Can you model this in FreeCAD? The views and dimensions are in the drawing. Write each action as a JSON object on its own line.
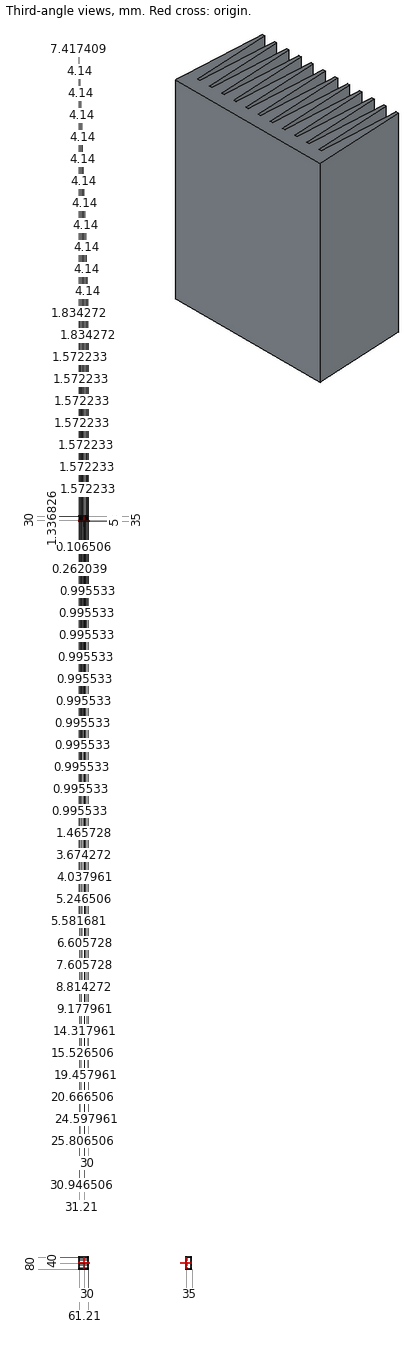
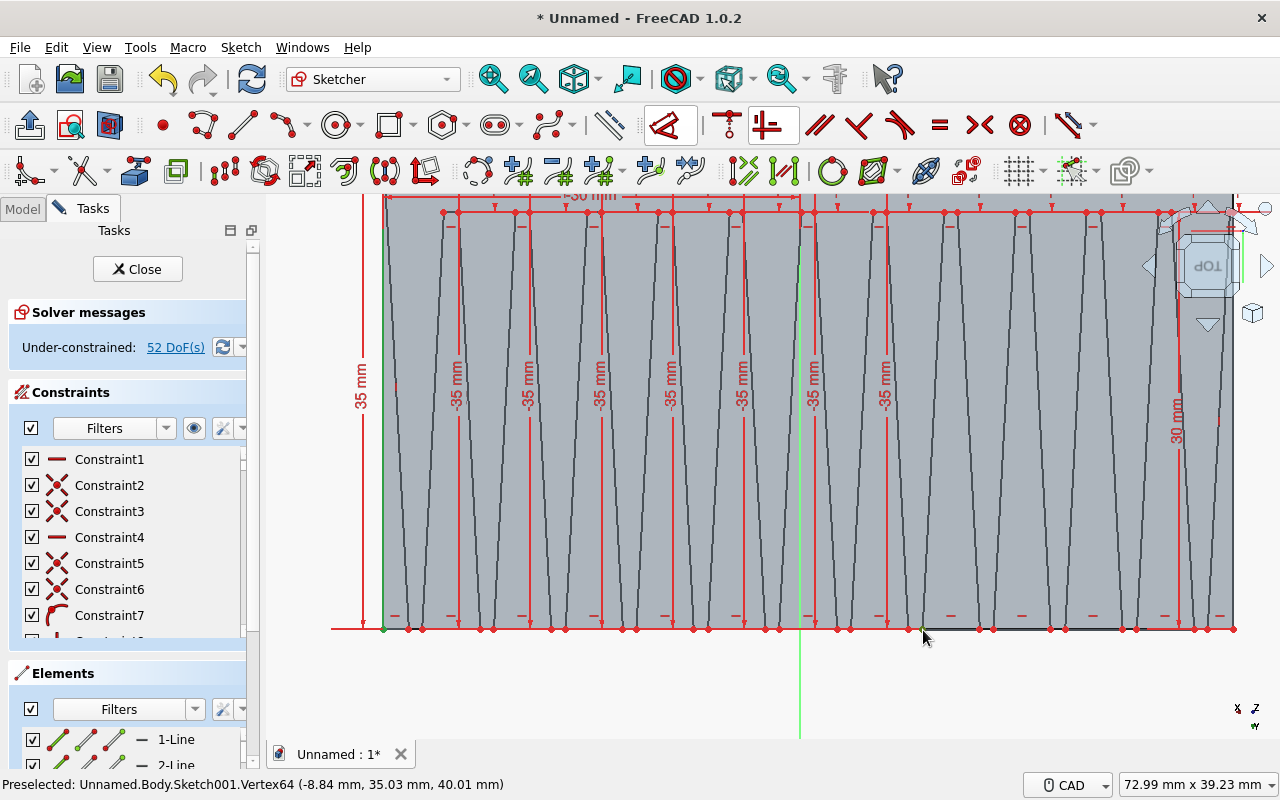
{"action": "left_click", "coordinate": [692, 126]}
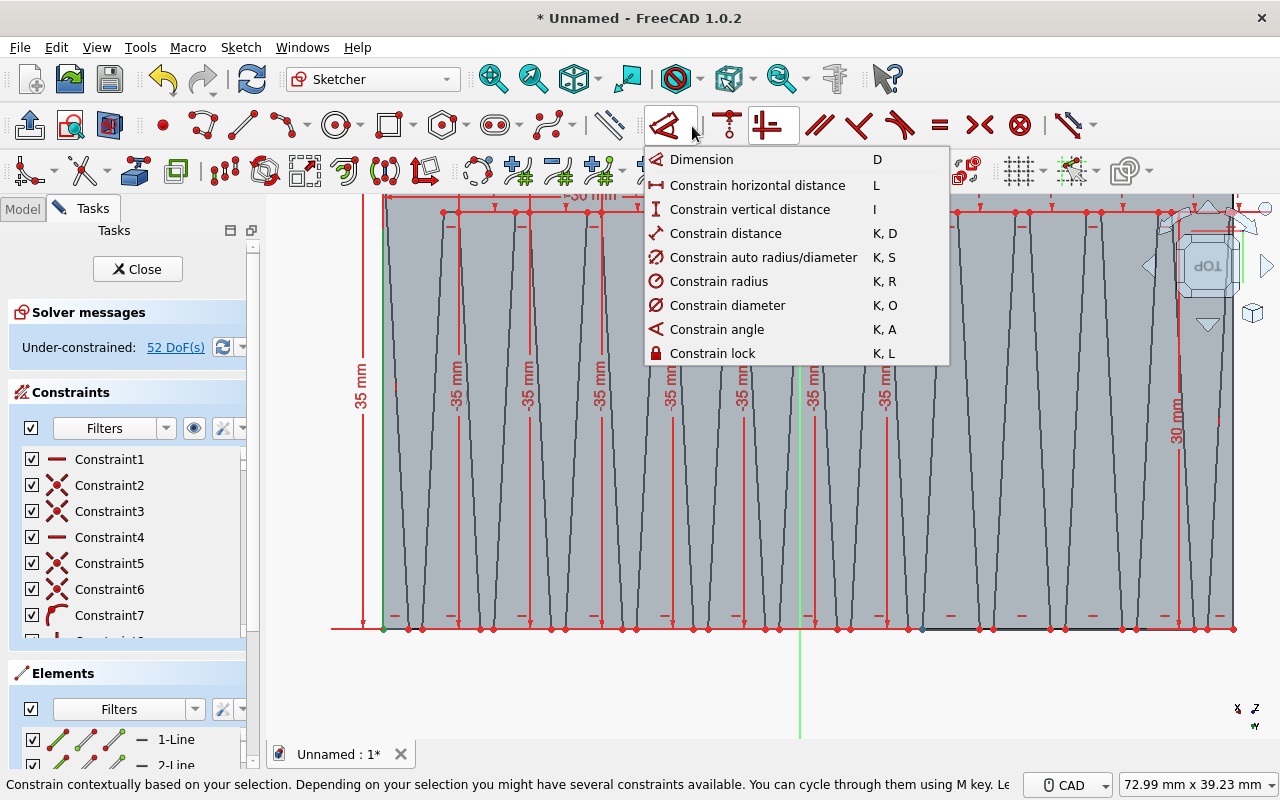
{"action": "left_click", "coordinate": [797, 209]}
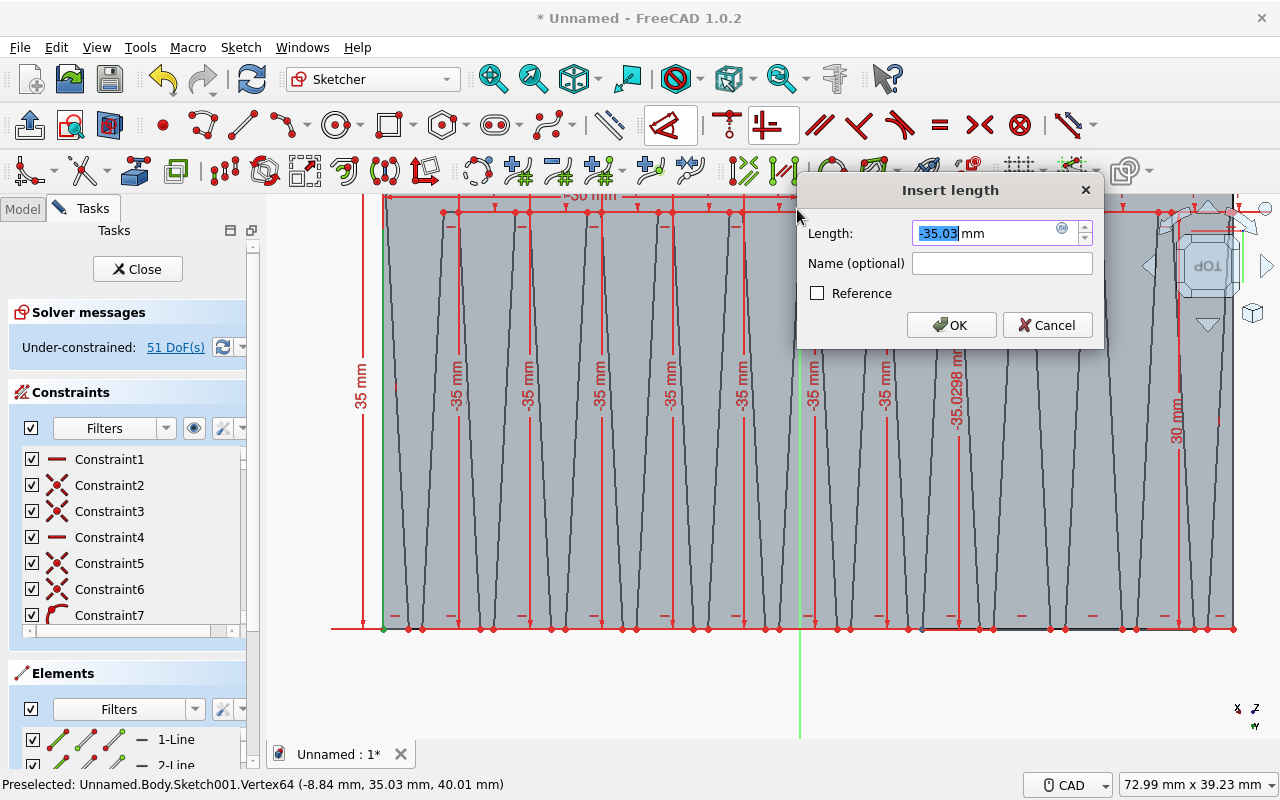
{"action": "type", "text": "-35"}
{"action": "key", "text": "Return"}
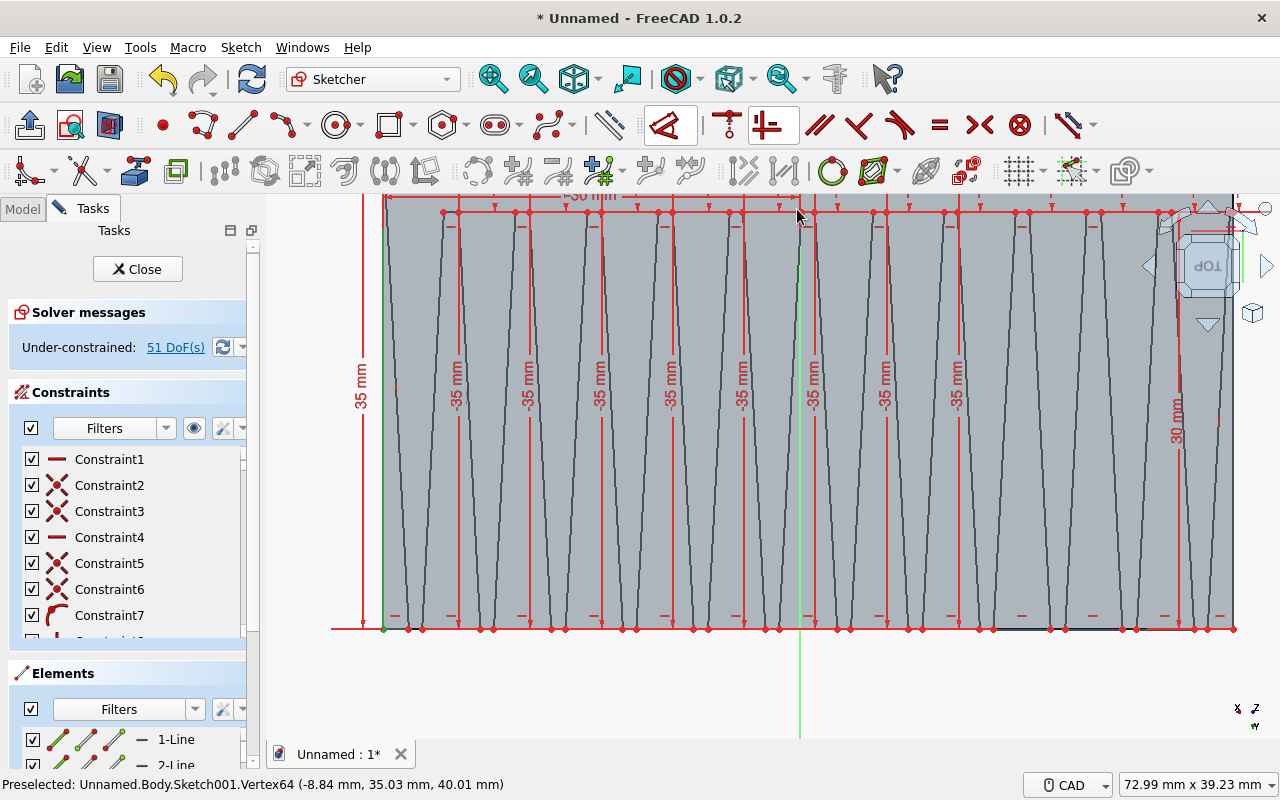
{"action": "left_click", "coordinate": [993, 630]}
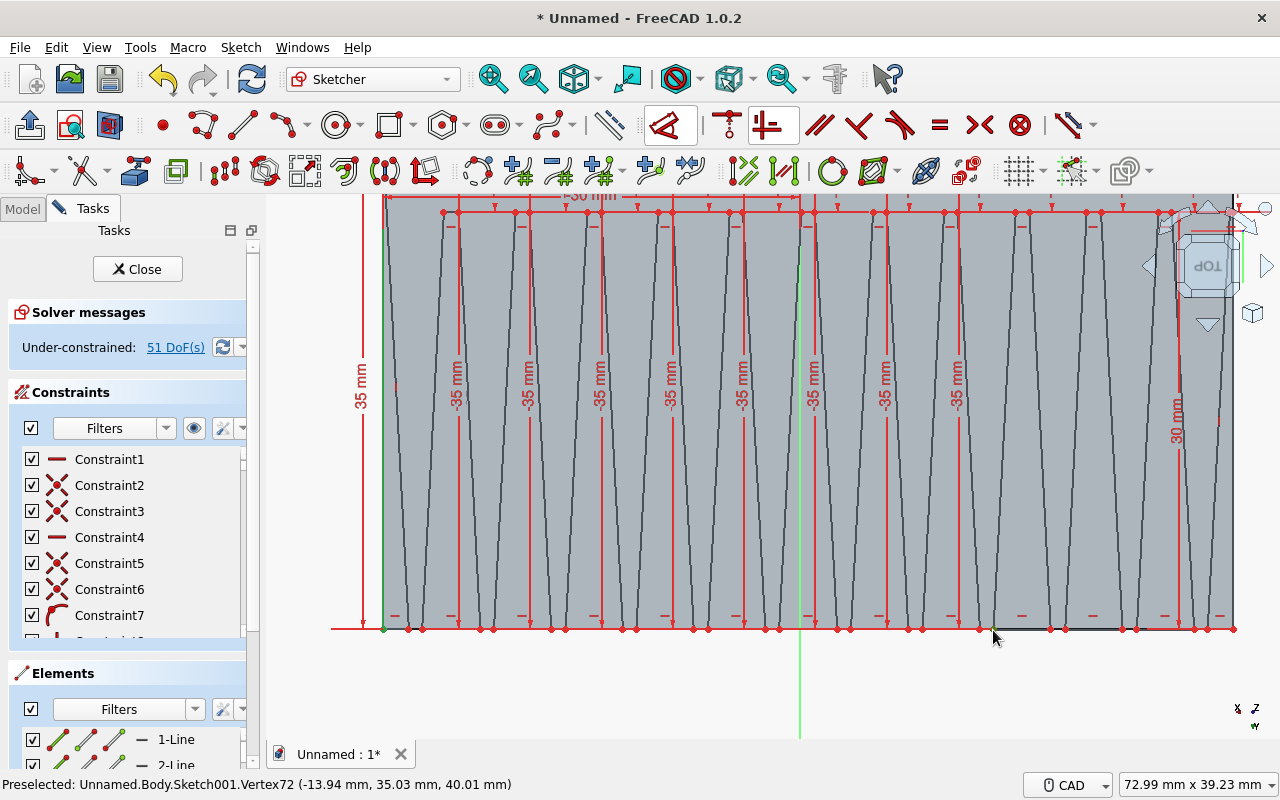
{"action": "left_click", "coordinate": [692, 126]}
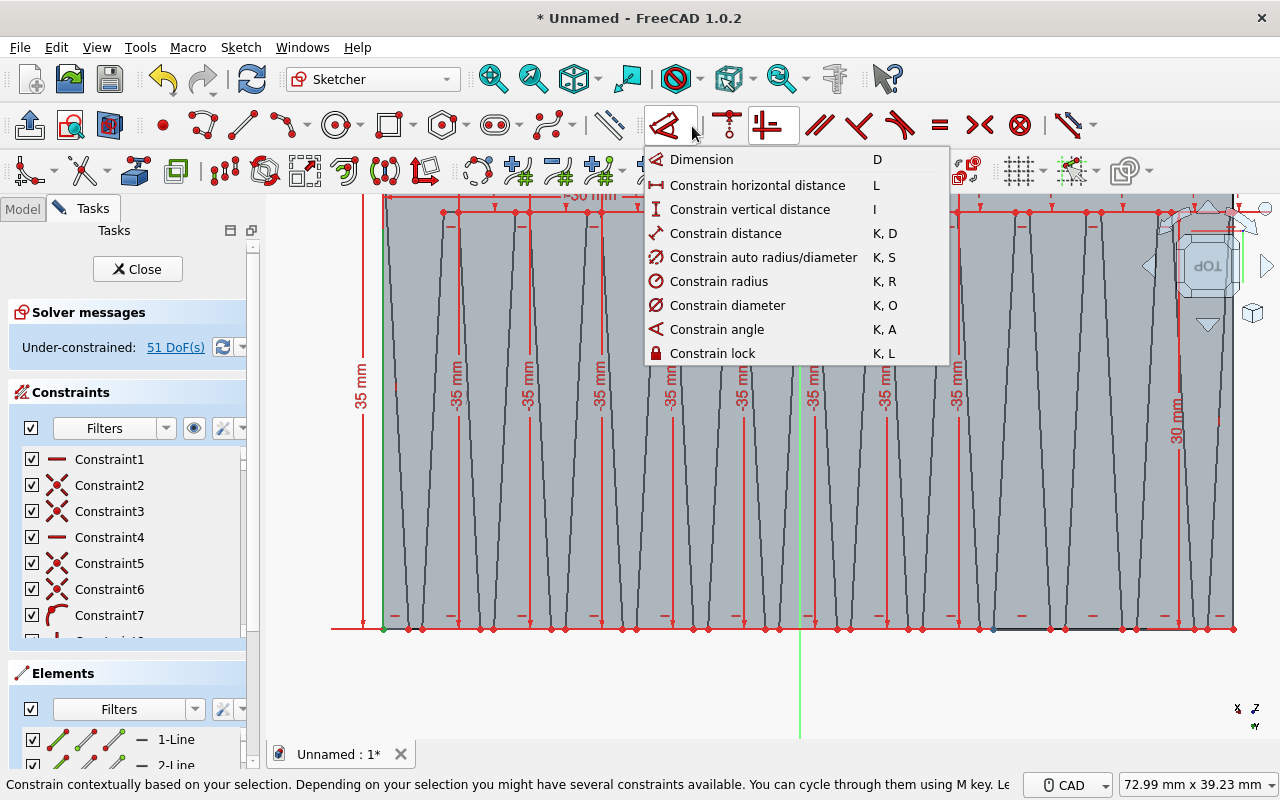
{"action": "left_click", "coordinate": [797, 209]}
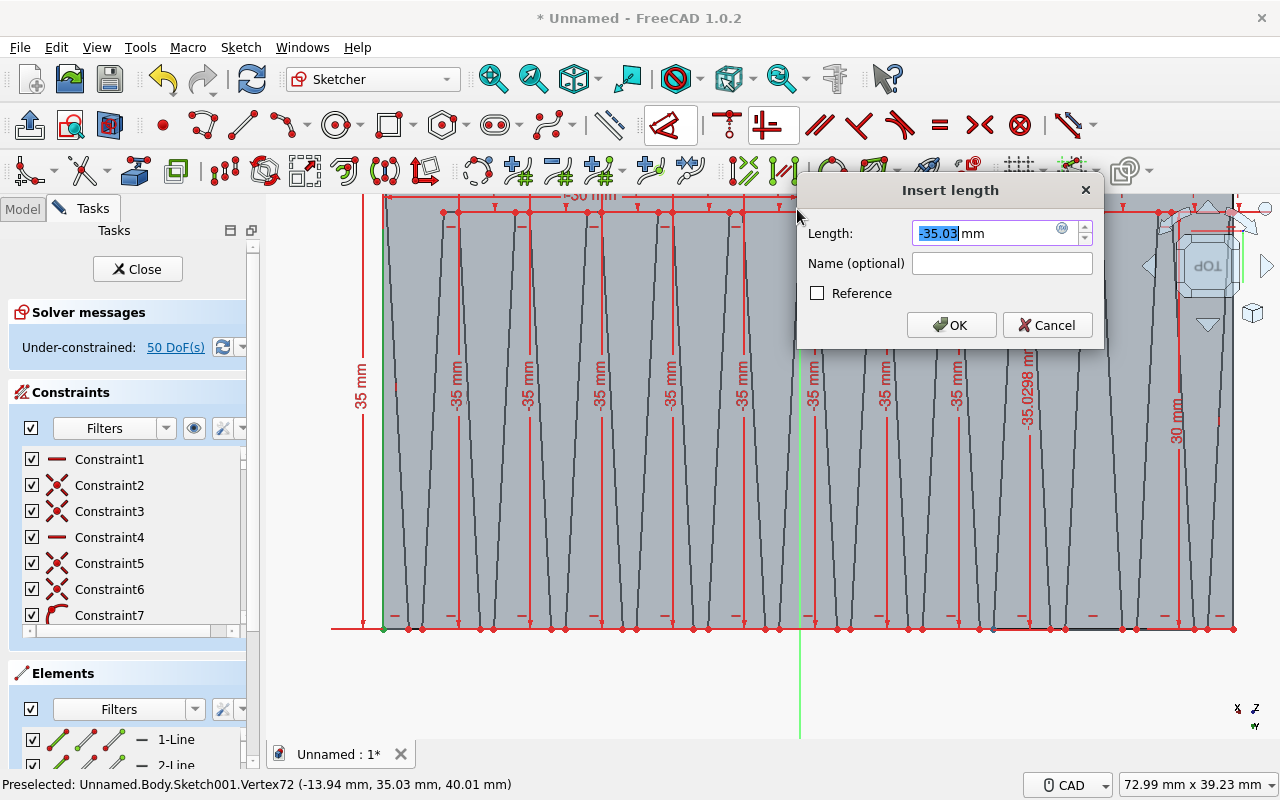
{"action": "type", "text": "-35"}
{"action": "key", "text": "Return"}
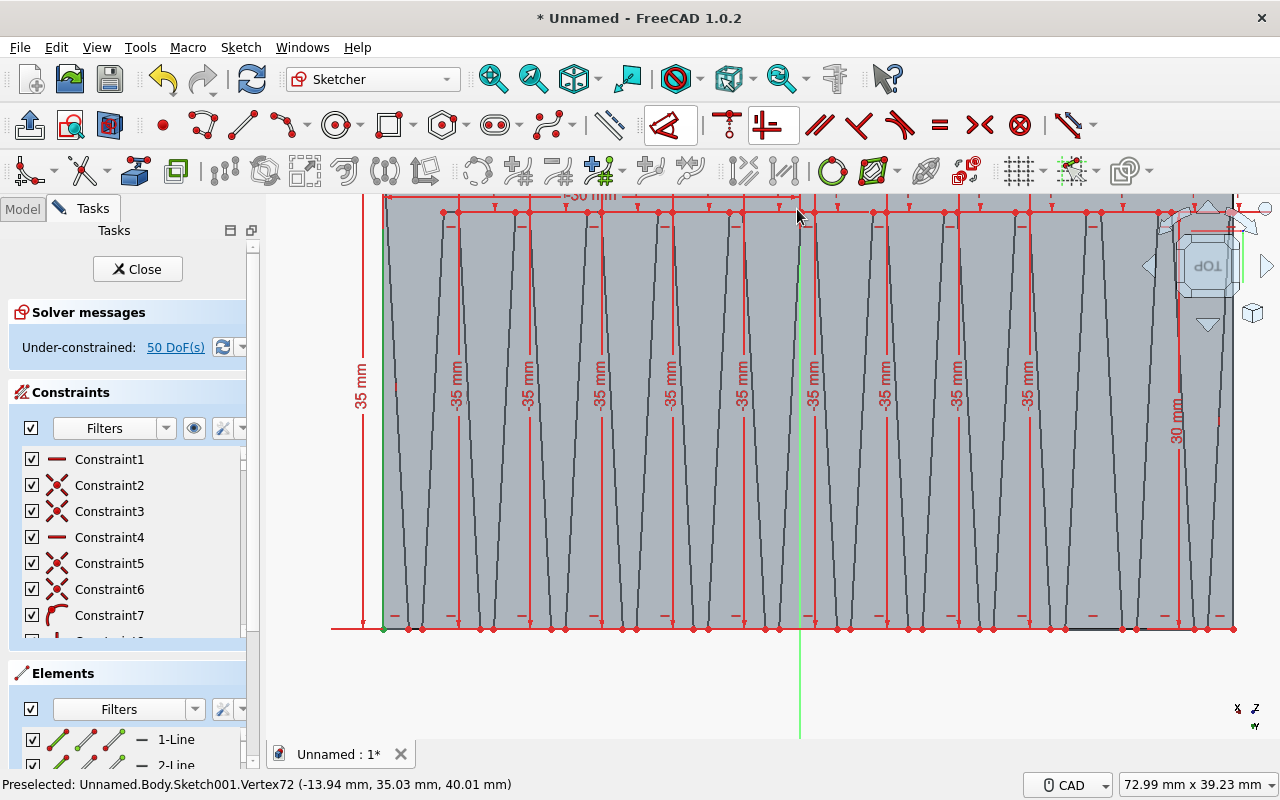
{"action": "left_click", "coordinate": [1065, 630]}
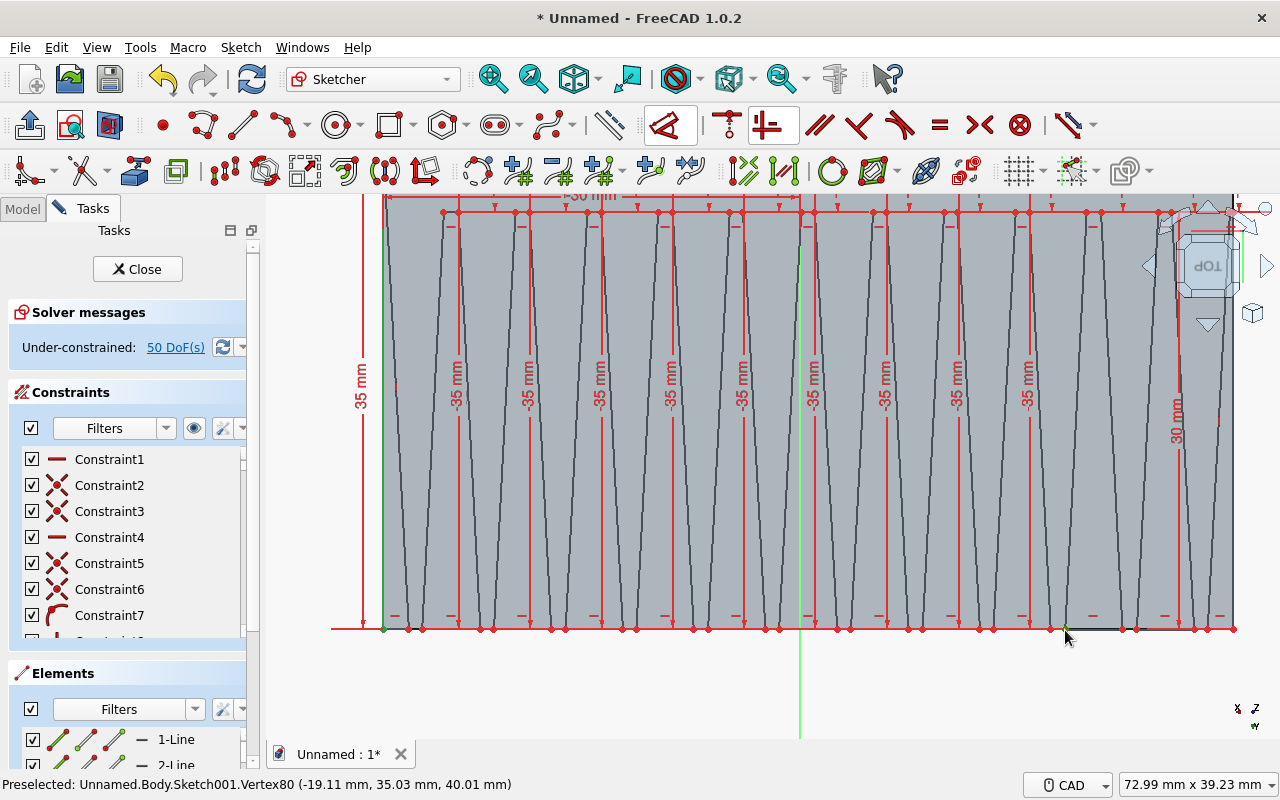
{"action": "key", "text": "i"}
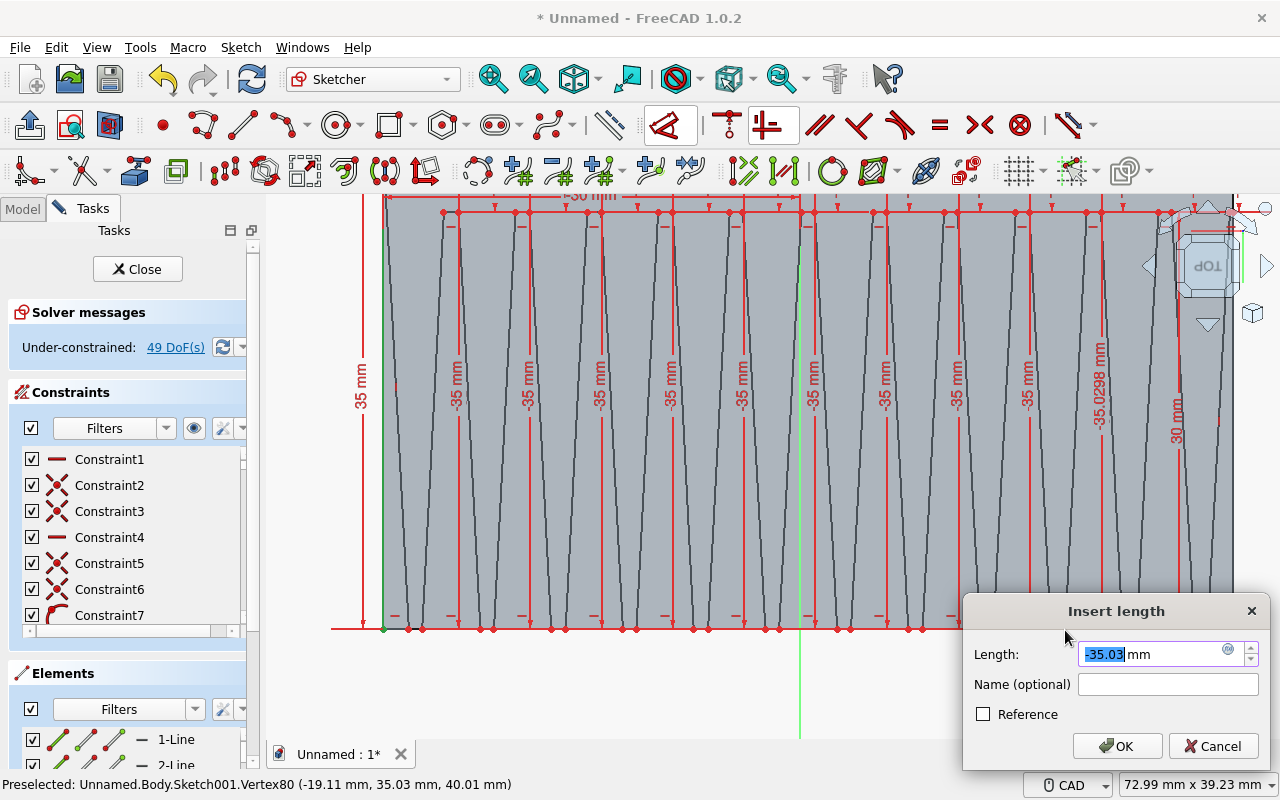
{"action": "type", "text": "-35"}
{"action": "key", "text": "Return"}